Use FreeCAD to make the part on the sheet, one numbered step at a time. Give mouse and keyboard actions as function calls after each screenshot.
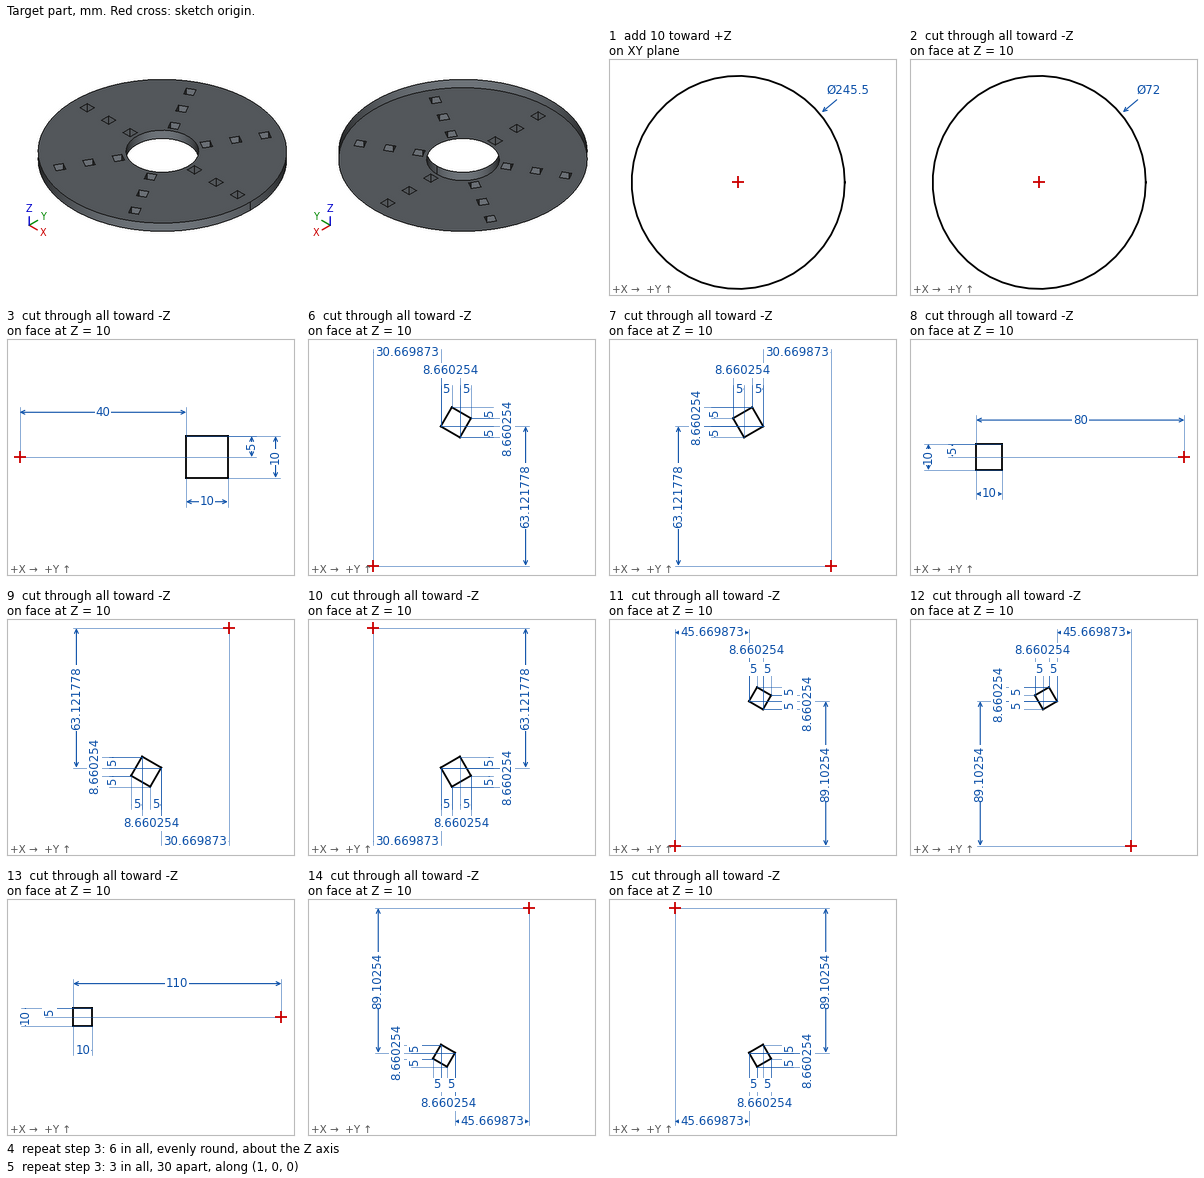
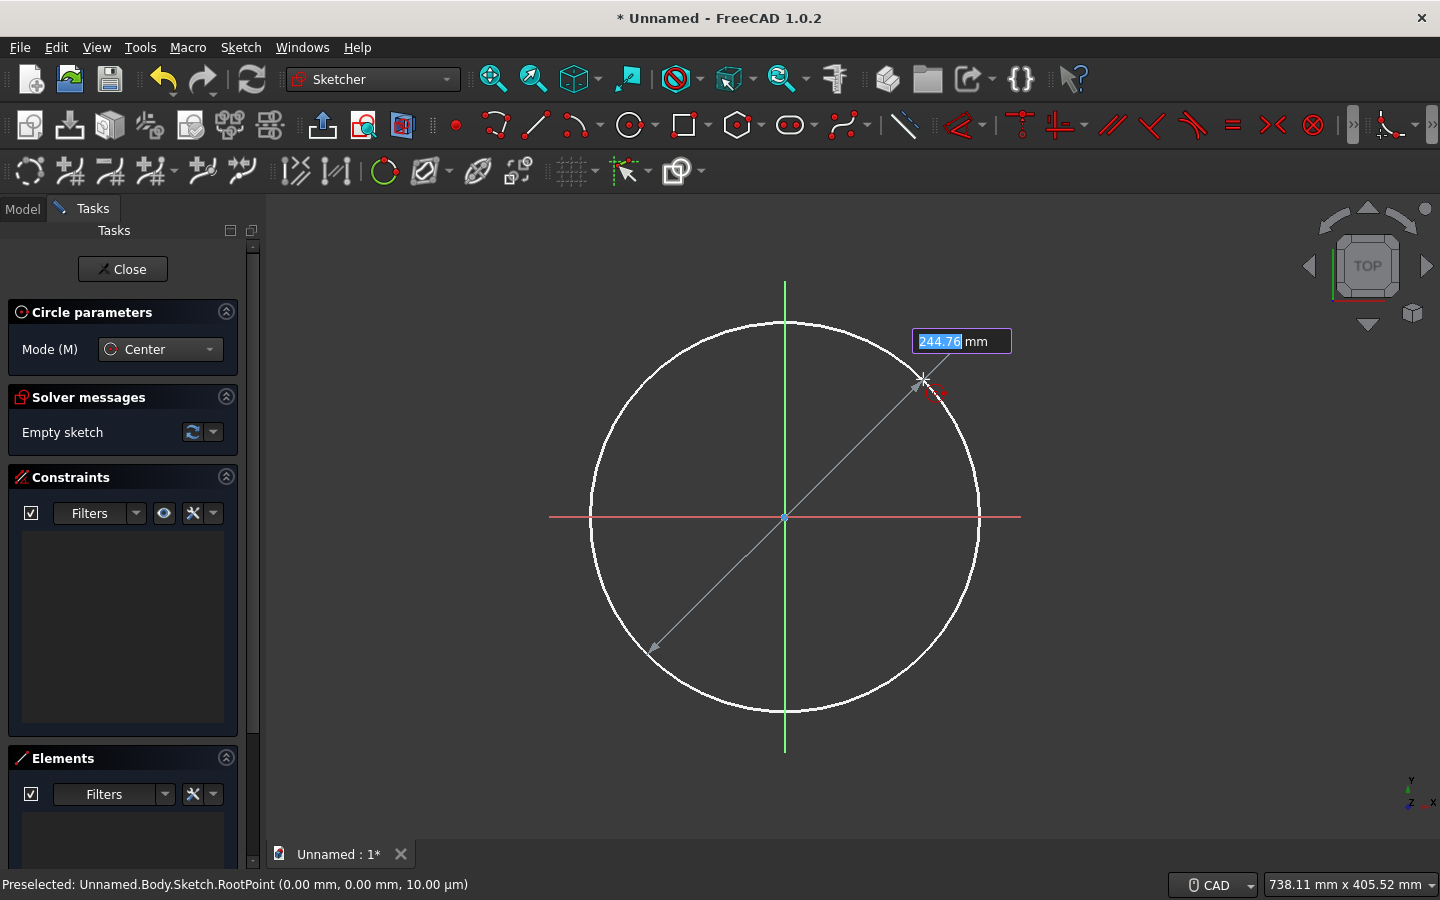
text(245.5)
key(Return)
key(Escape)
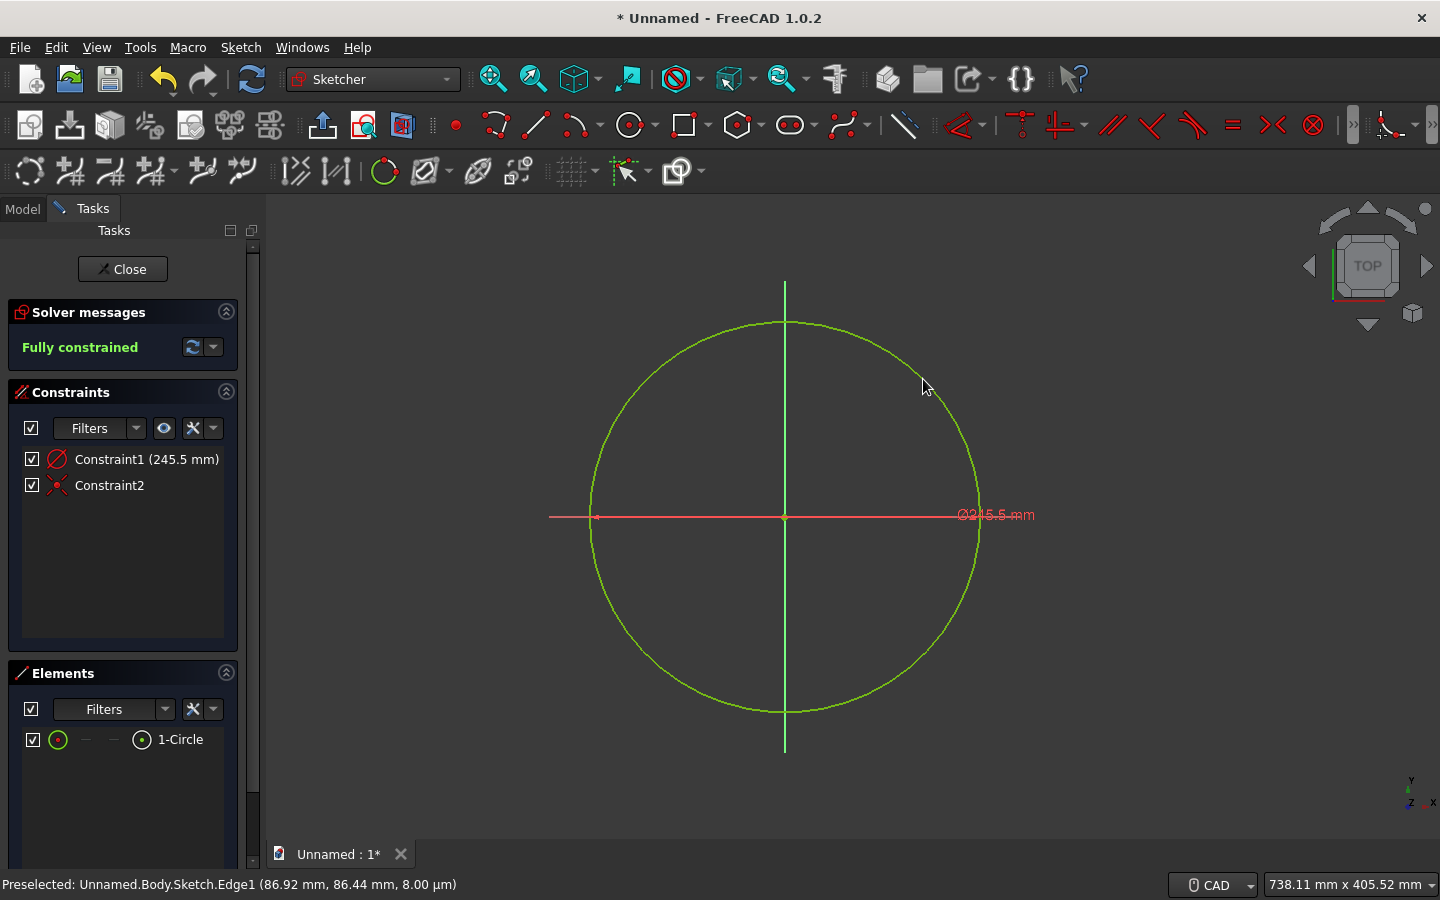
click(123, 269)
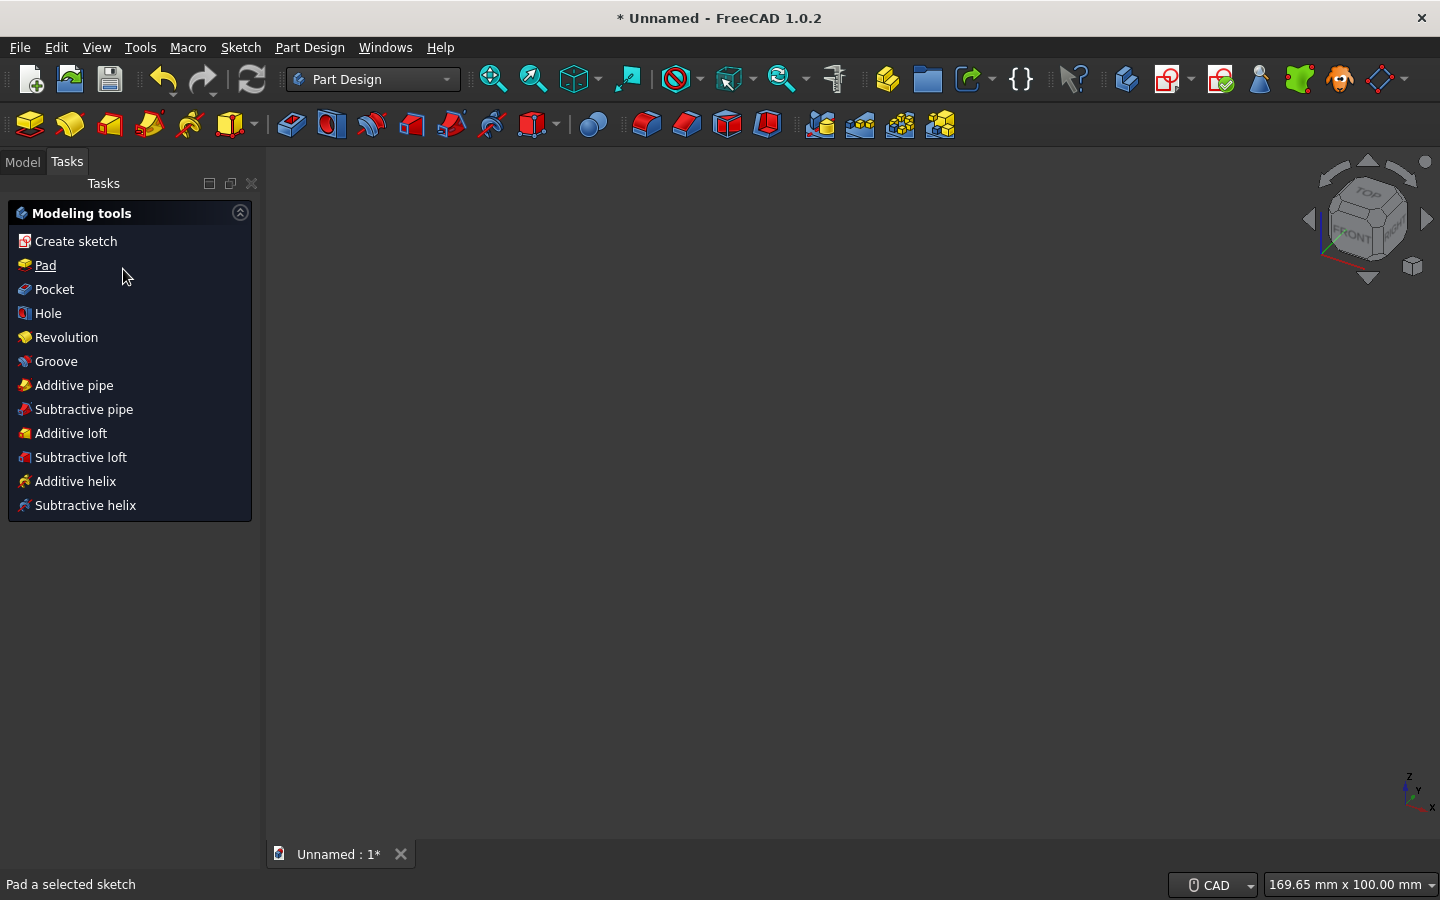
click(30, 124)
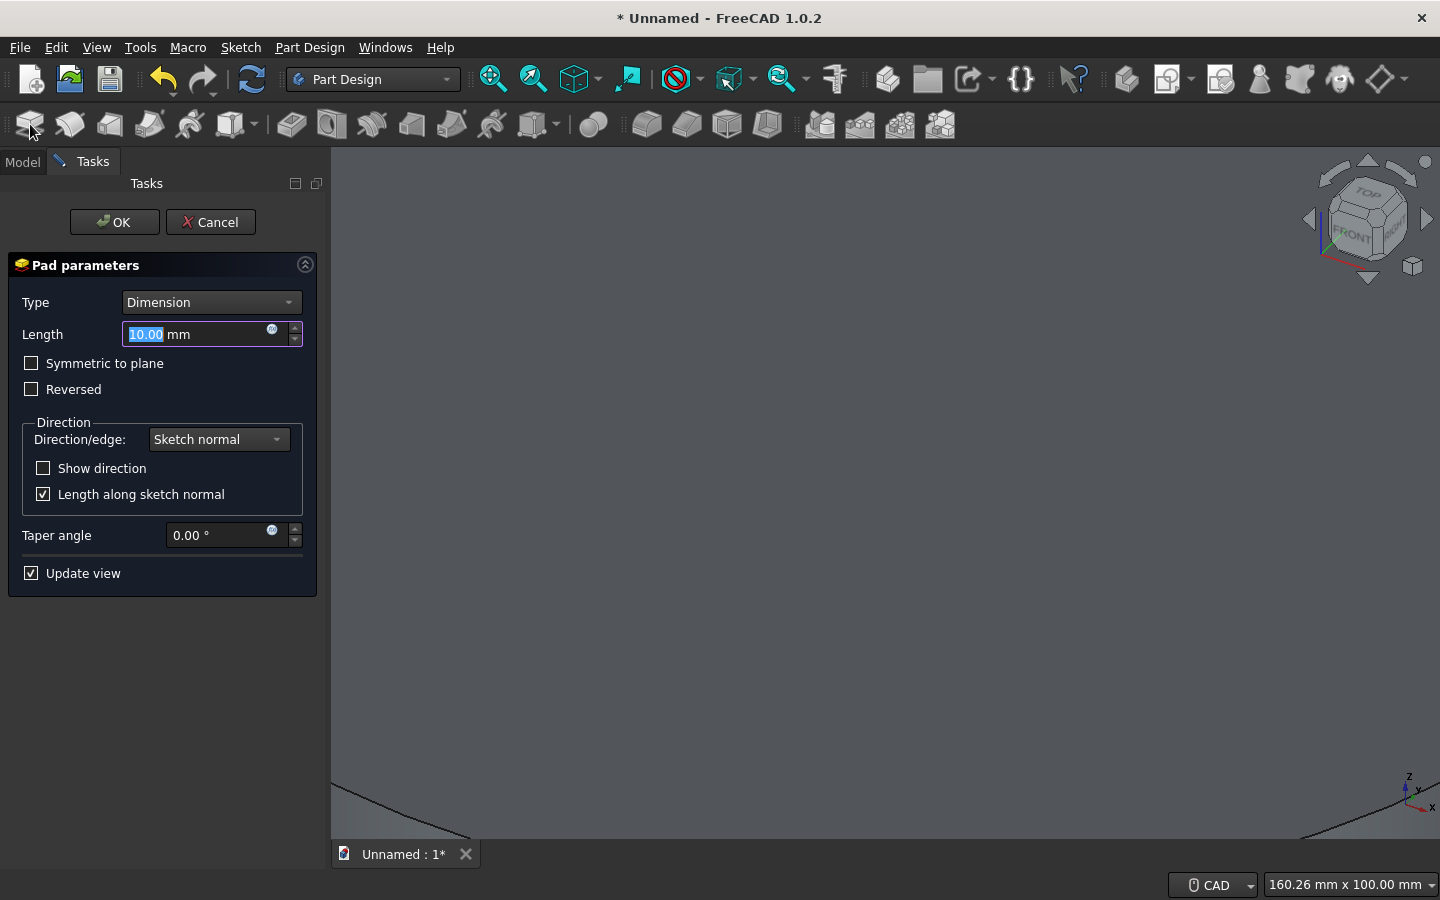
text(10)
key(Tab)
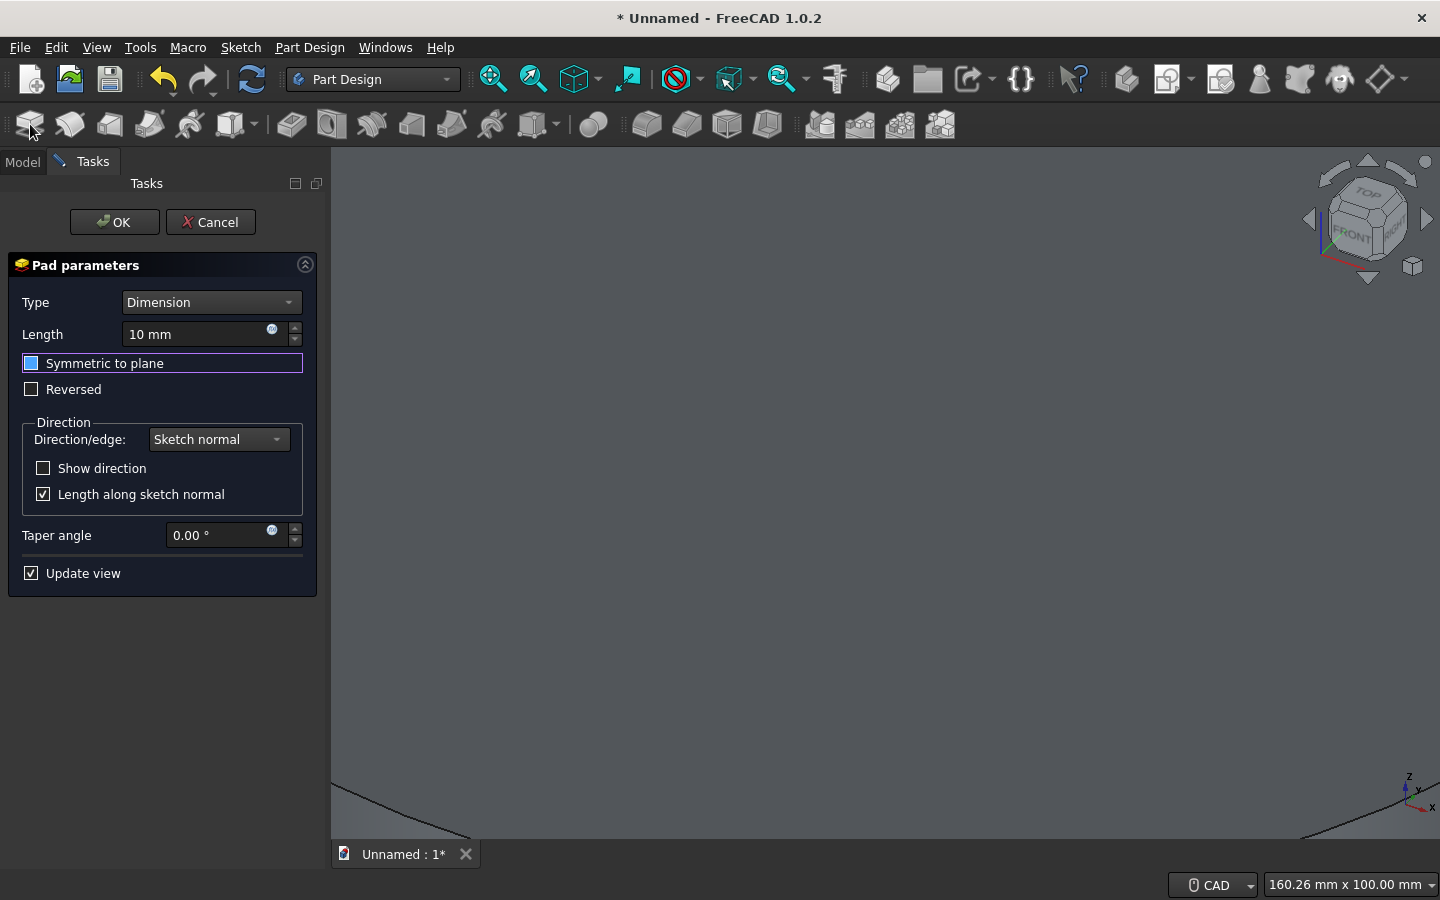
click(115, 222)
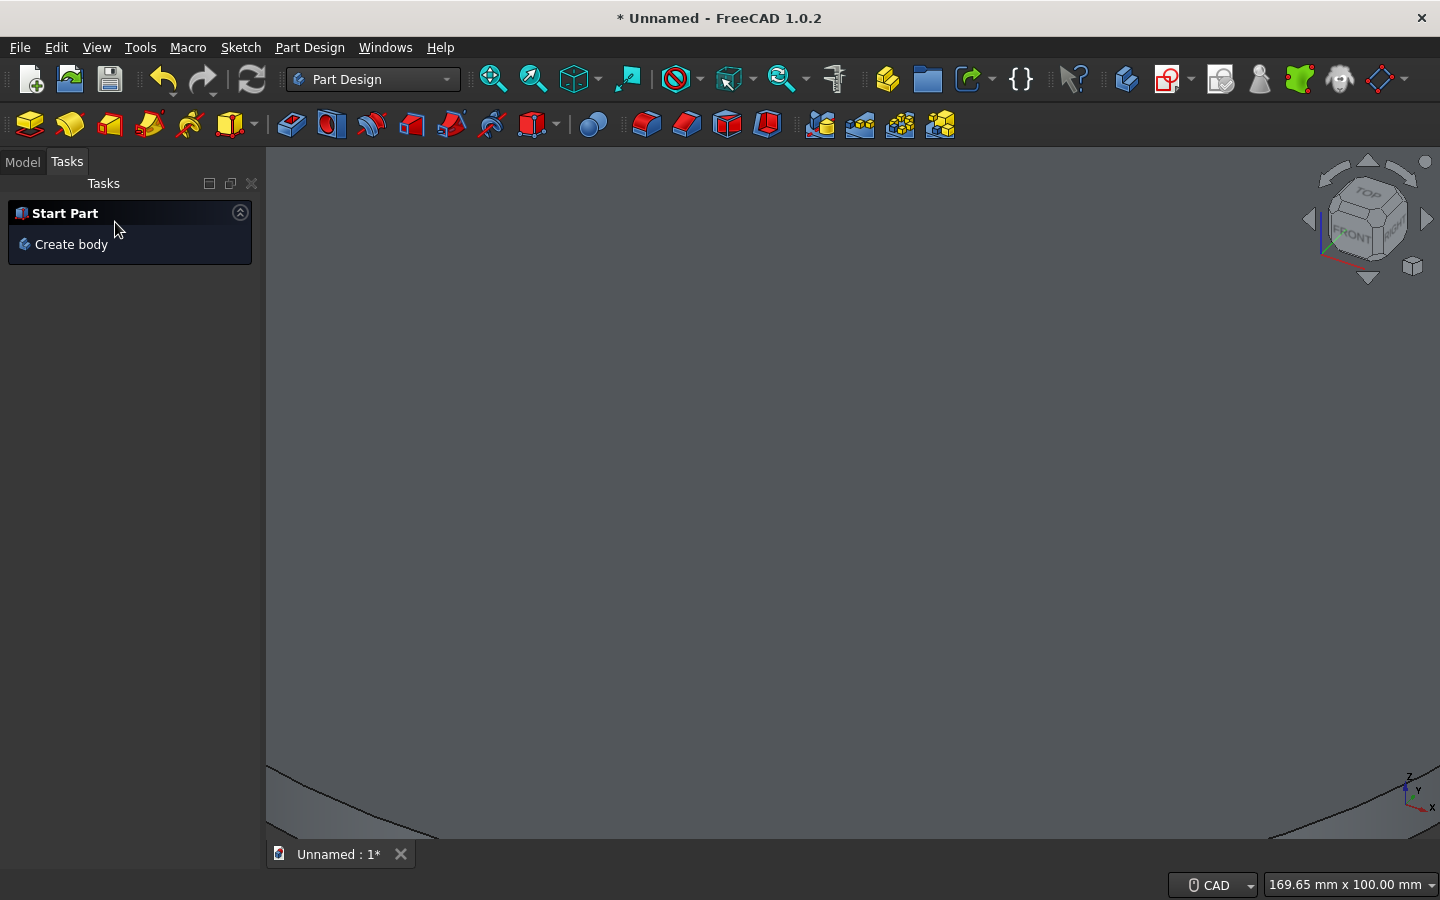
click(494, 80)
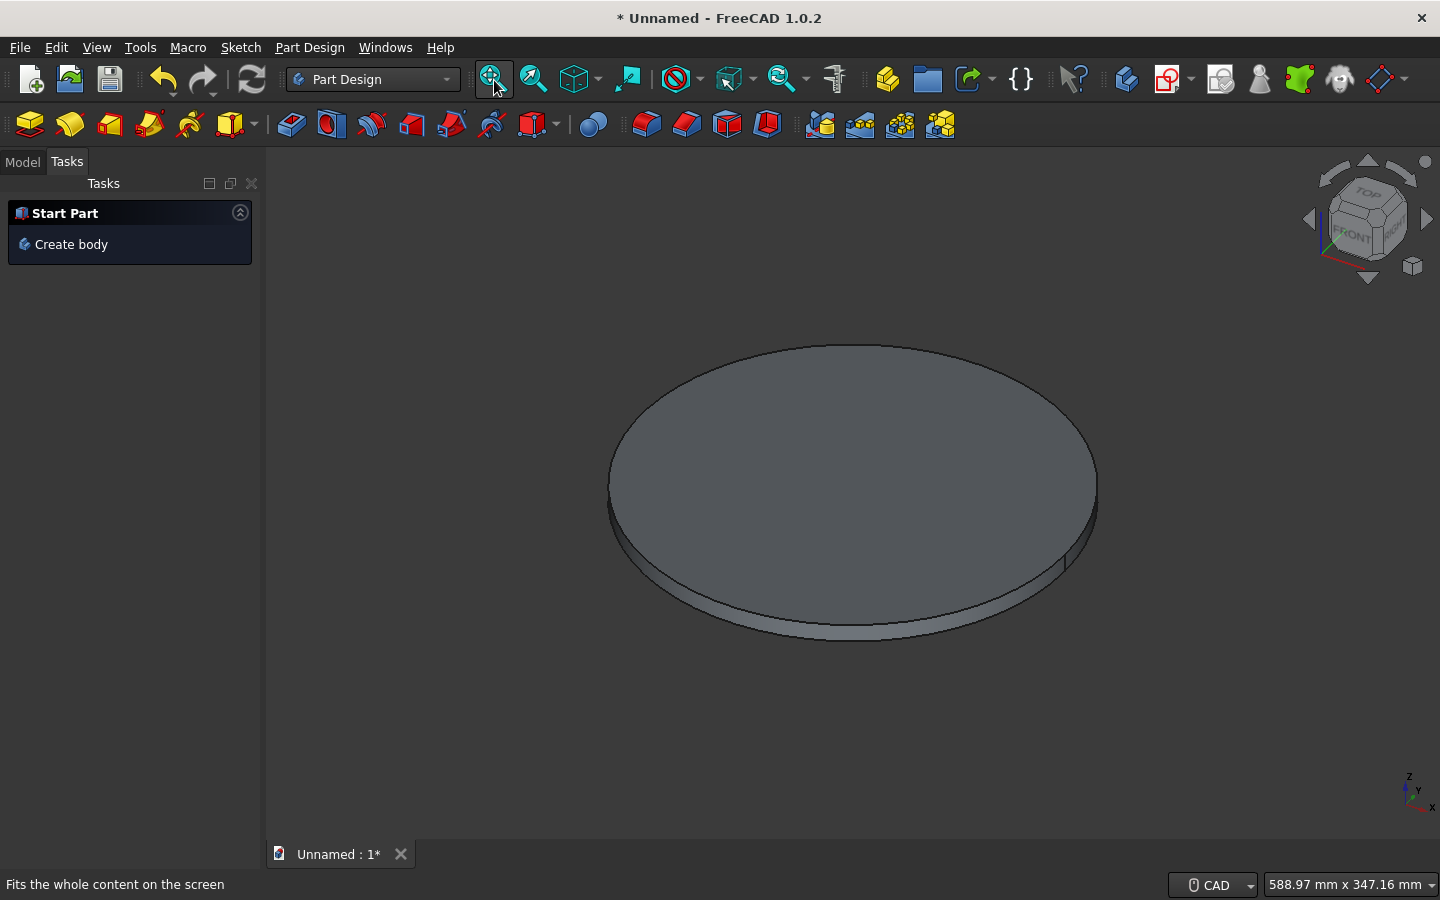
click(853, 484)